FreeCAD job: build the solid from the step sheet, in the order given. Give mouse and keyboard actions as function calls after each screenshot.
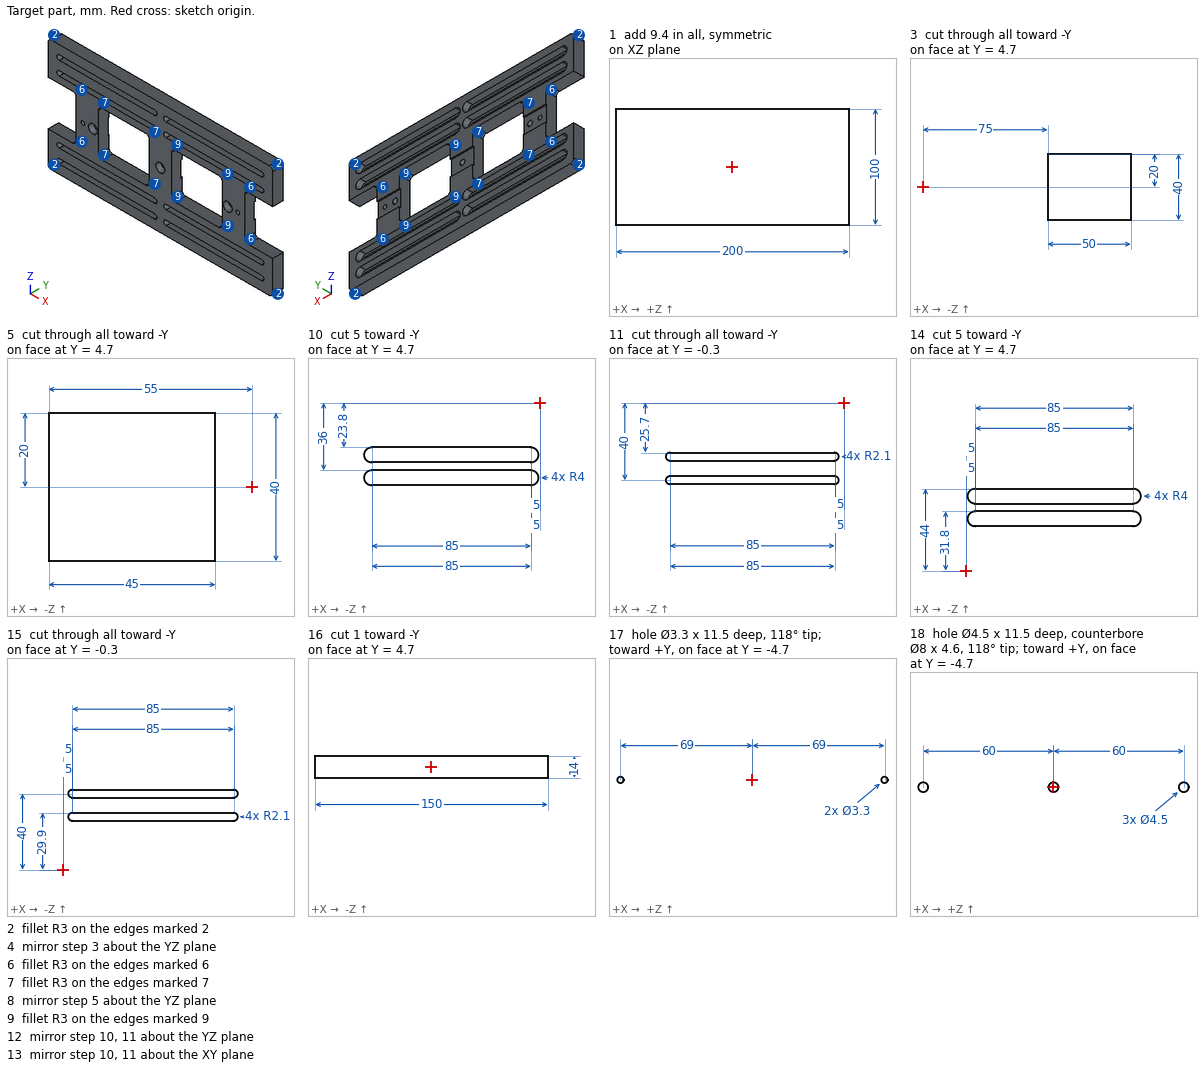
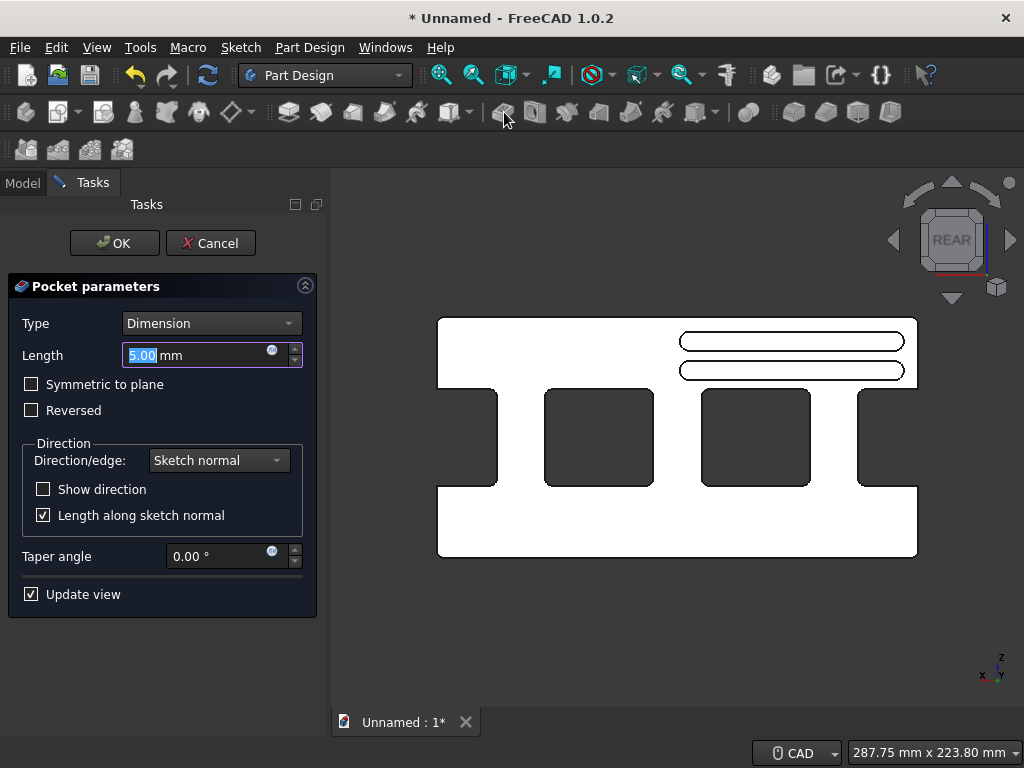
text(5)
key(Tab)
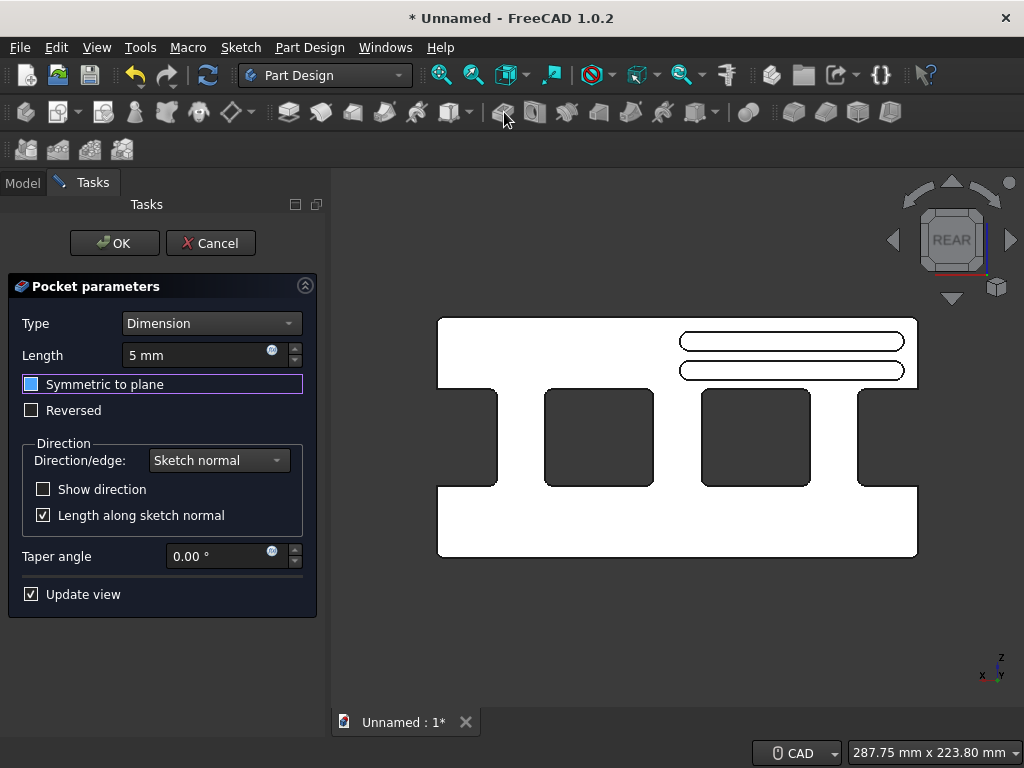
click(115, 243)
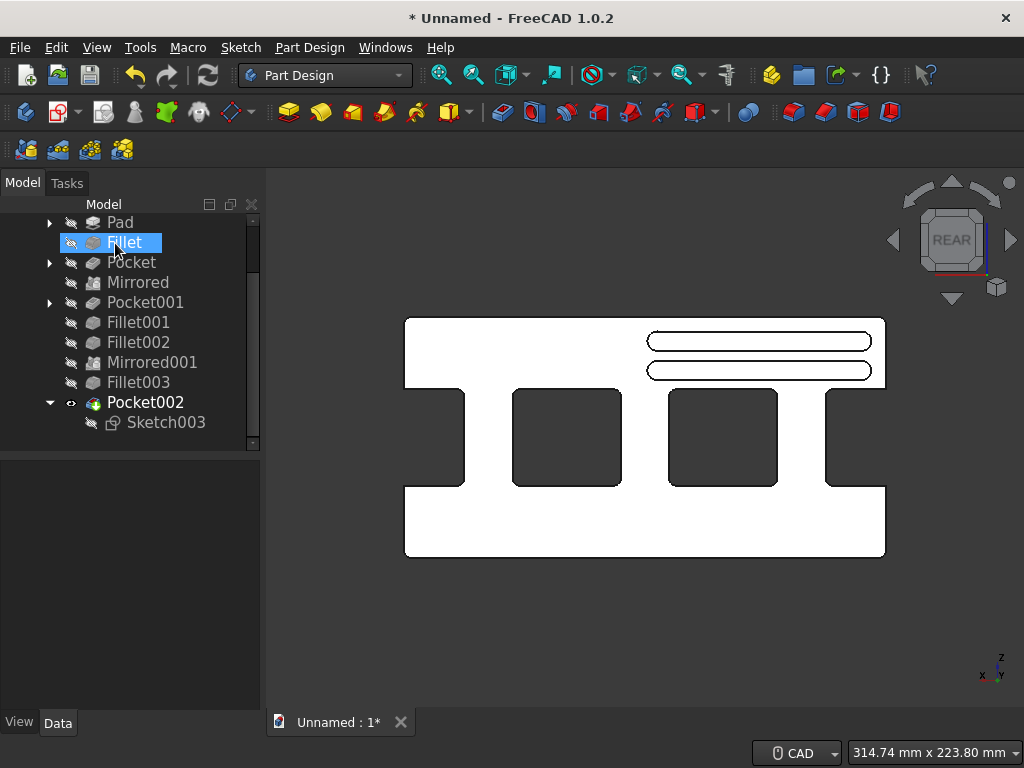
click(663, 370)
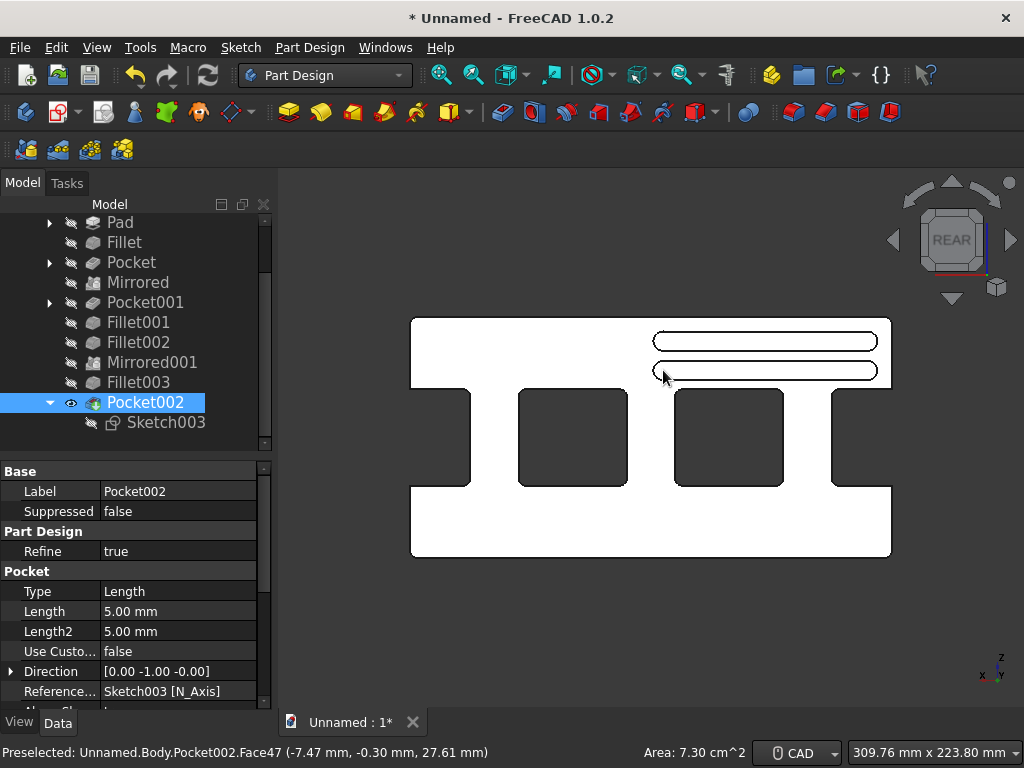
click(58, 112)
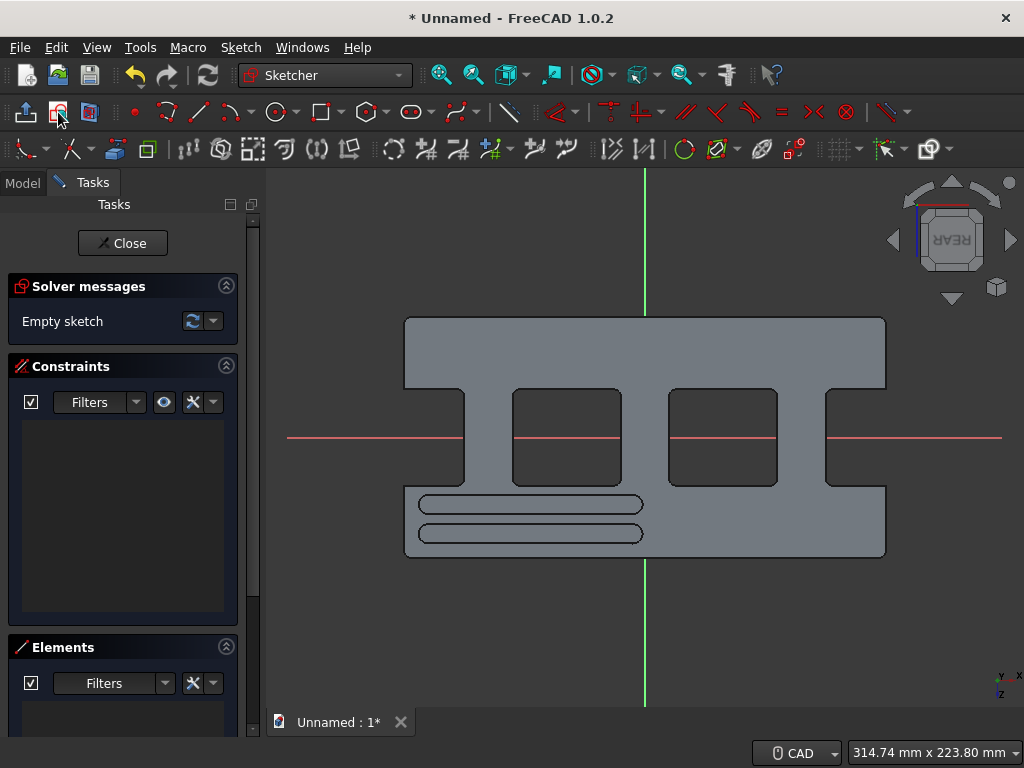
scroll(483, 550, up, 3)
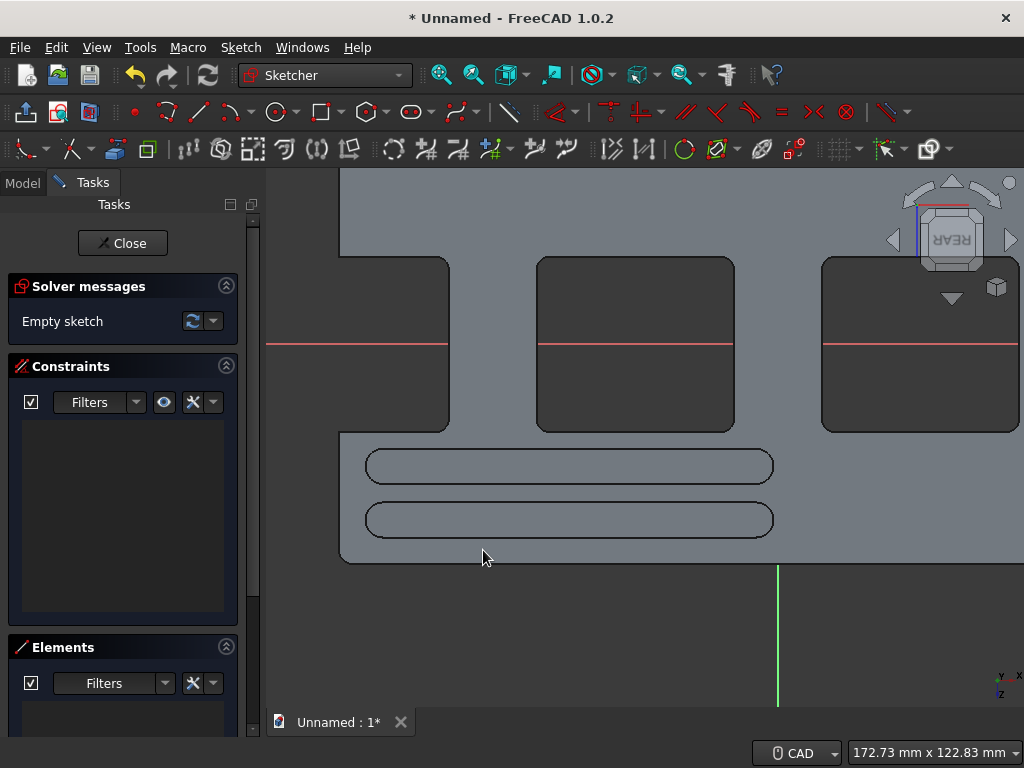
key(g)
key(s)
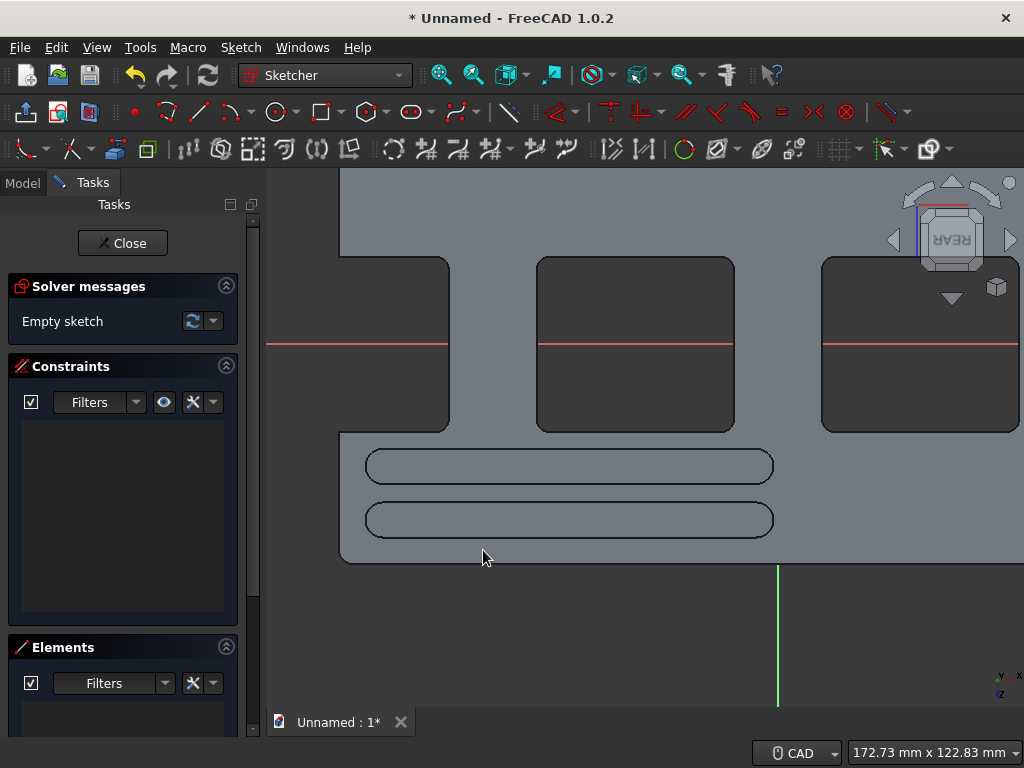
scroll(383, 466, up, 5)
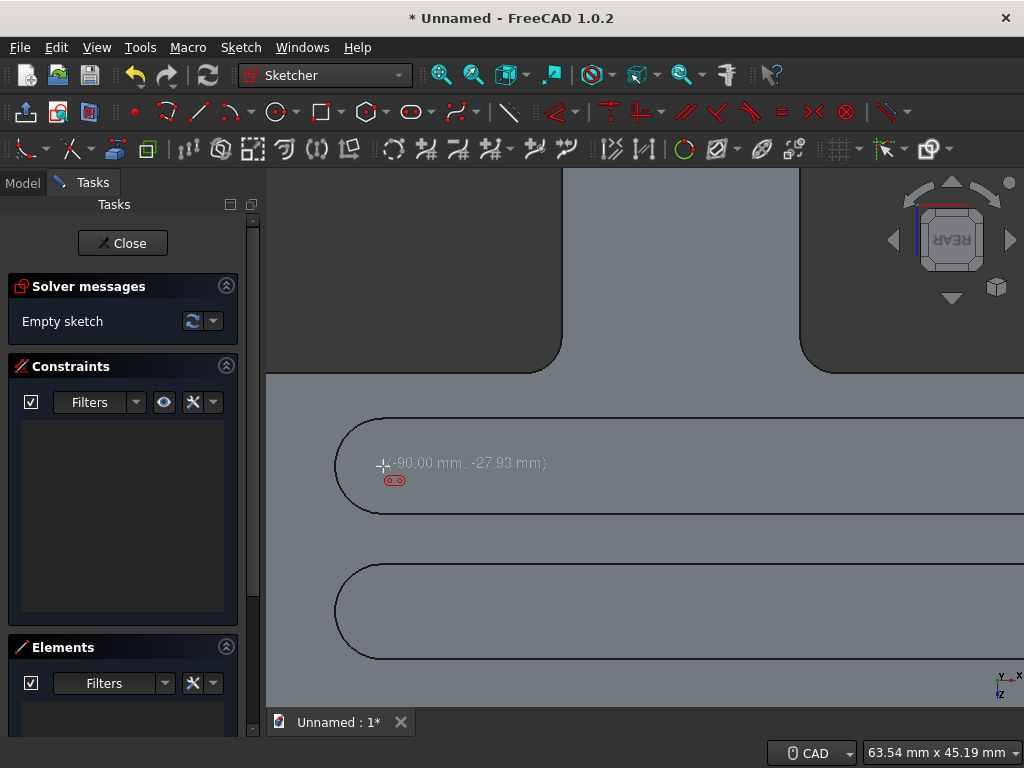
click(383, 466)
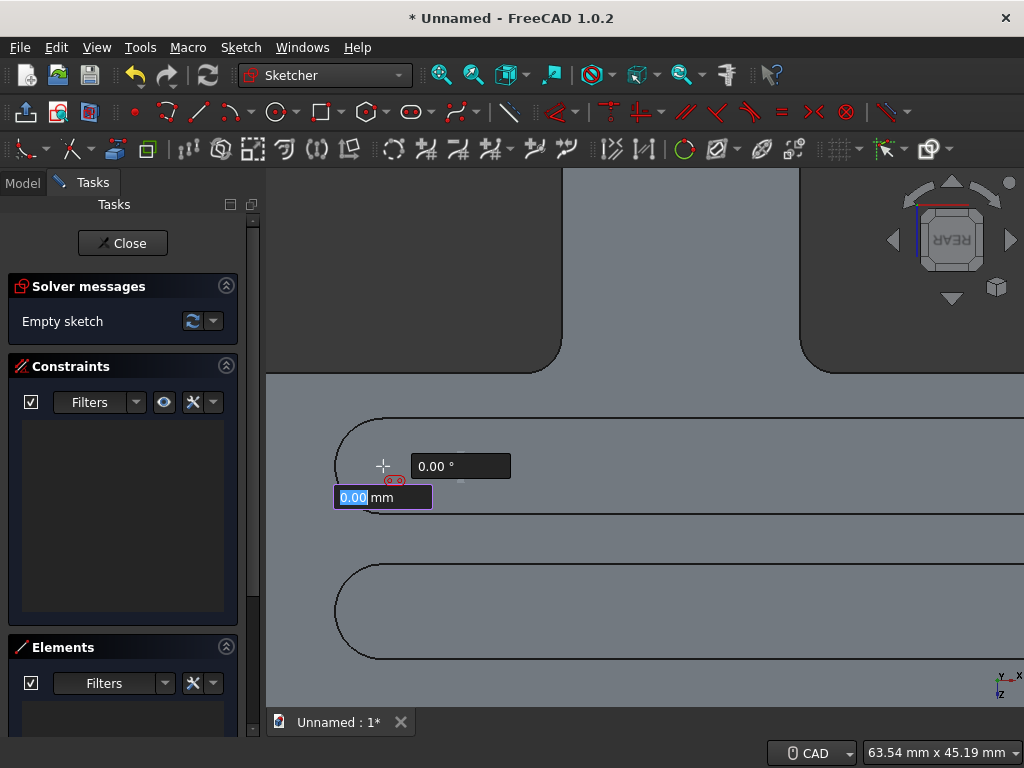
scroll(384, 468, down, 5)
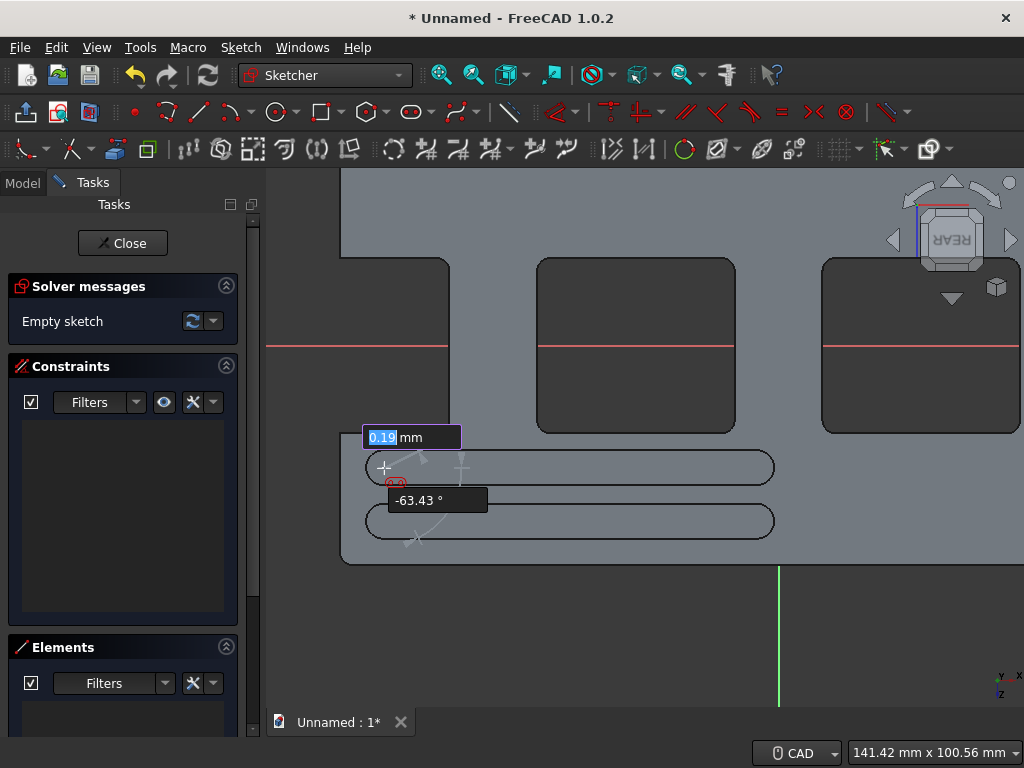
click(757, 468)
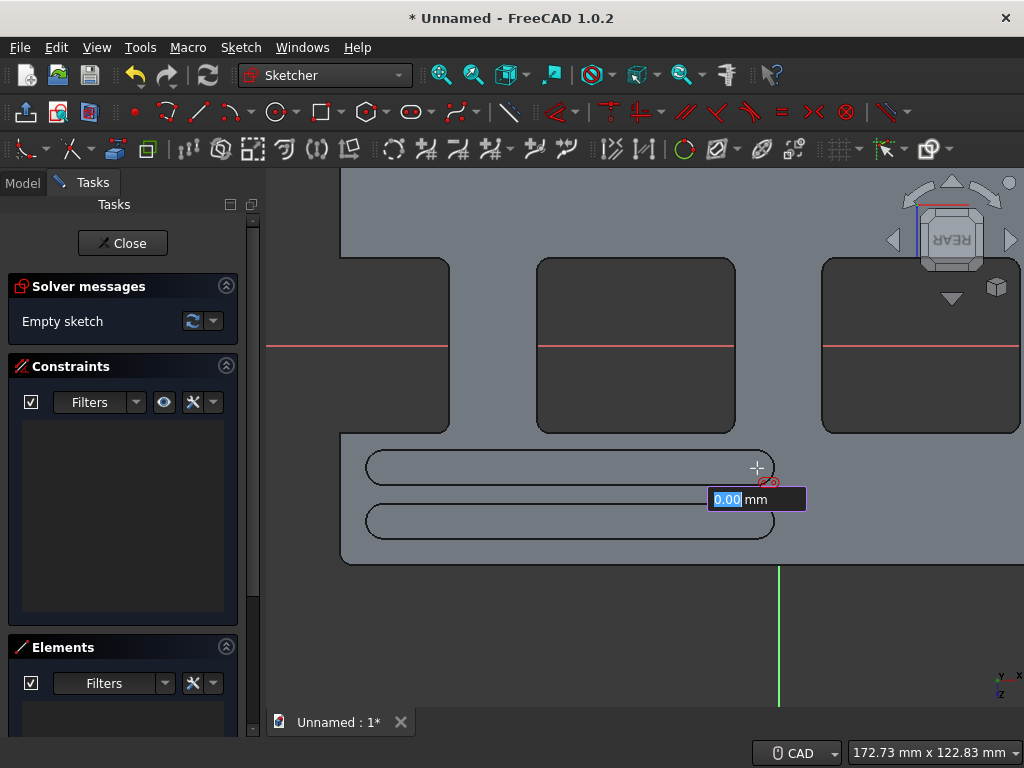
scroll(570, 458, up, 3)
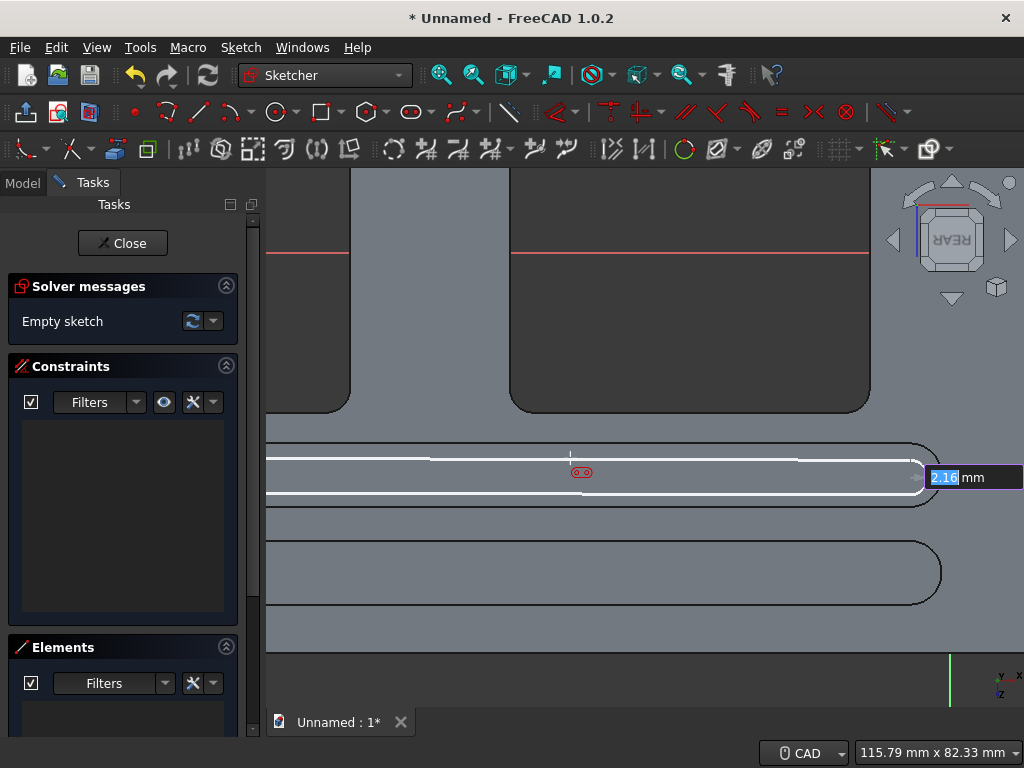
click(570, 458)